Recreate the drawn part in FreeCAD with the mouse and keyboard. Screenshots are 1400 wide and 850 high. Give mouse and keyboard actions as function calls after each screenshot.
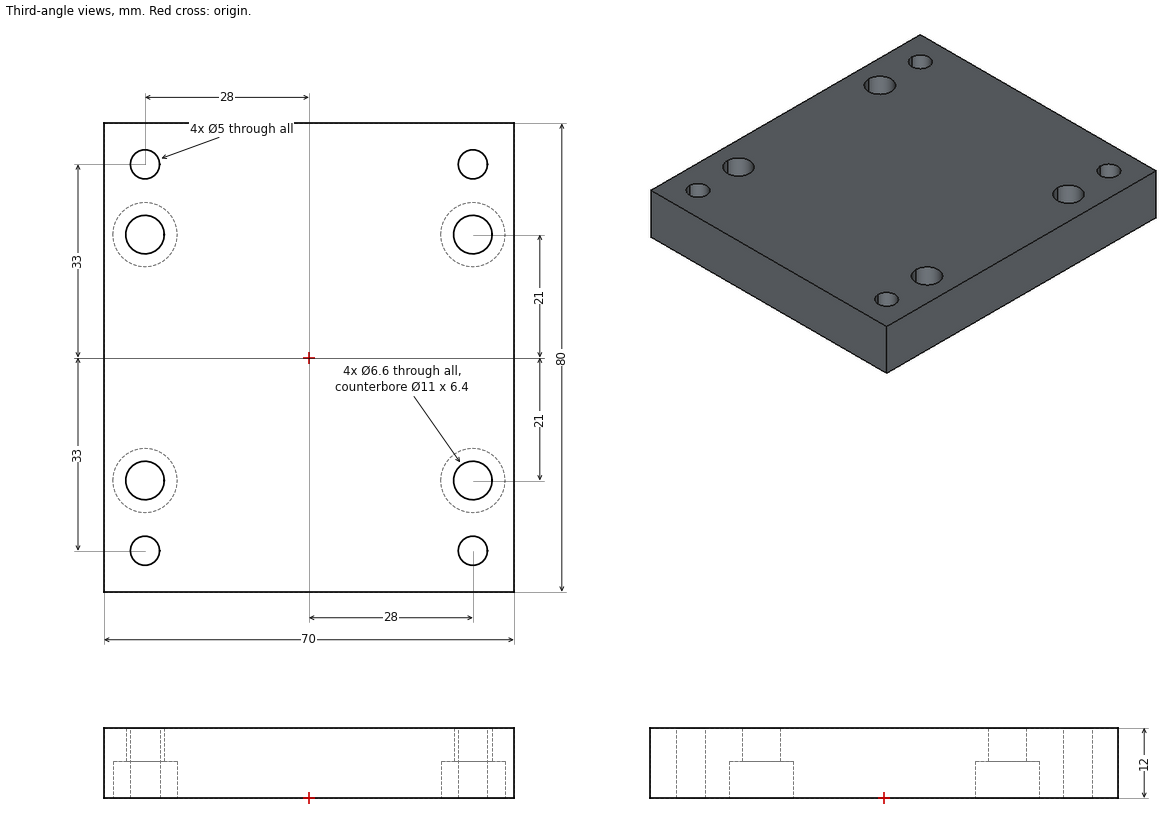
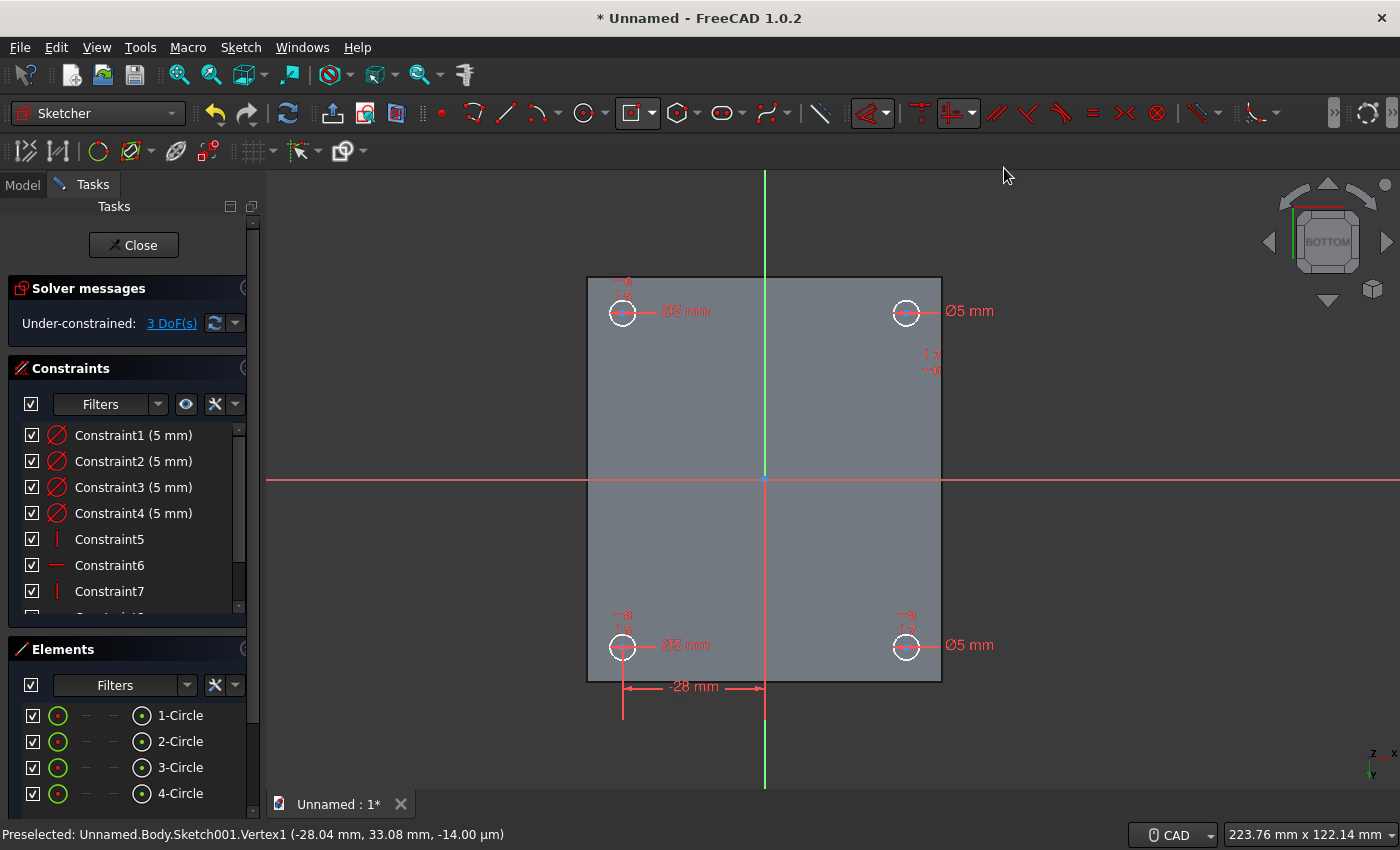
click(623, 647)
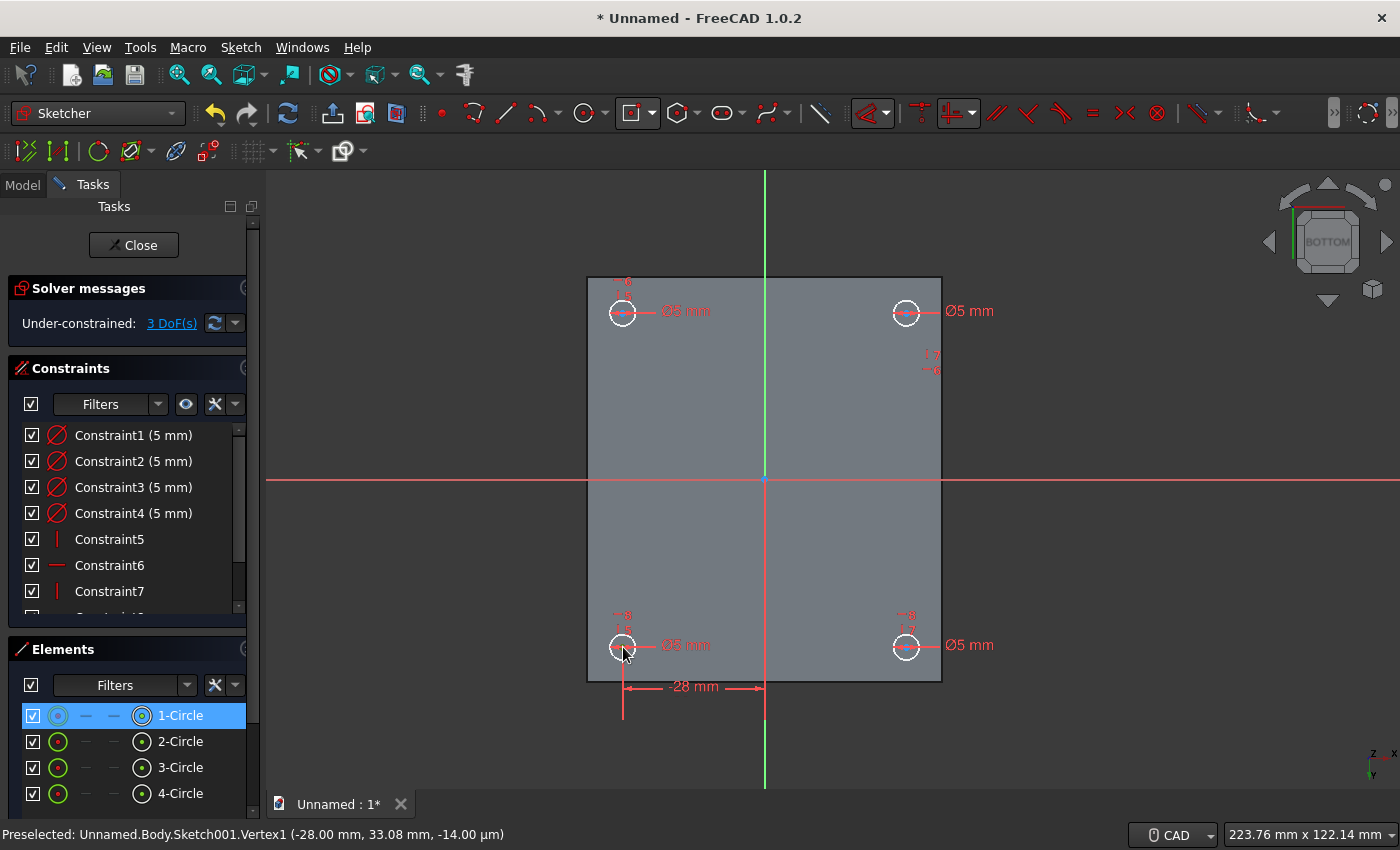
click(888, 114)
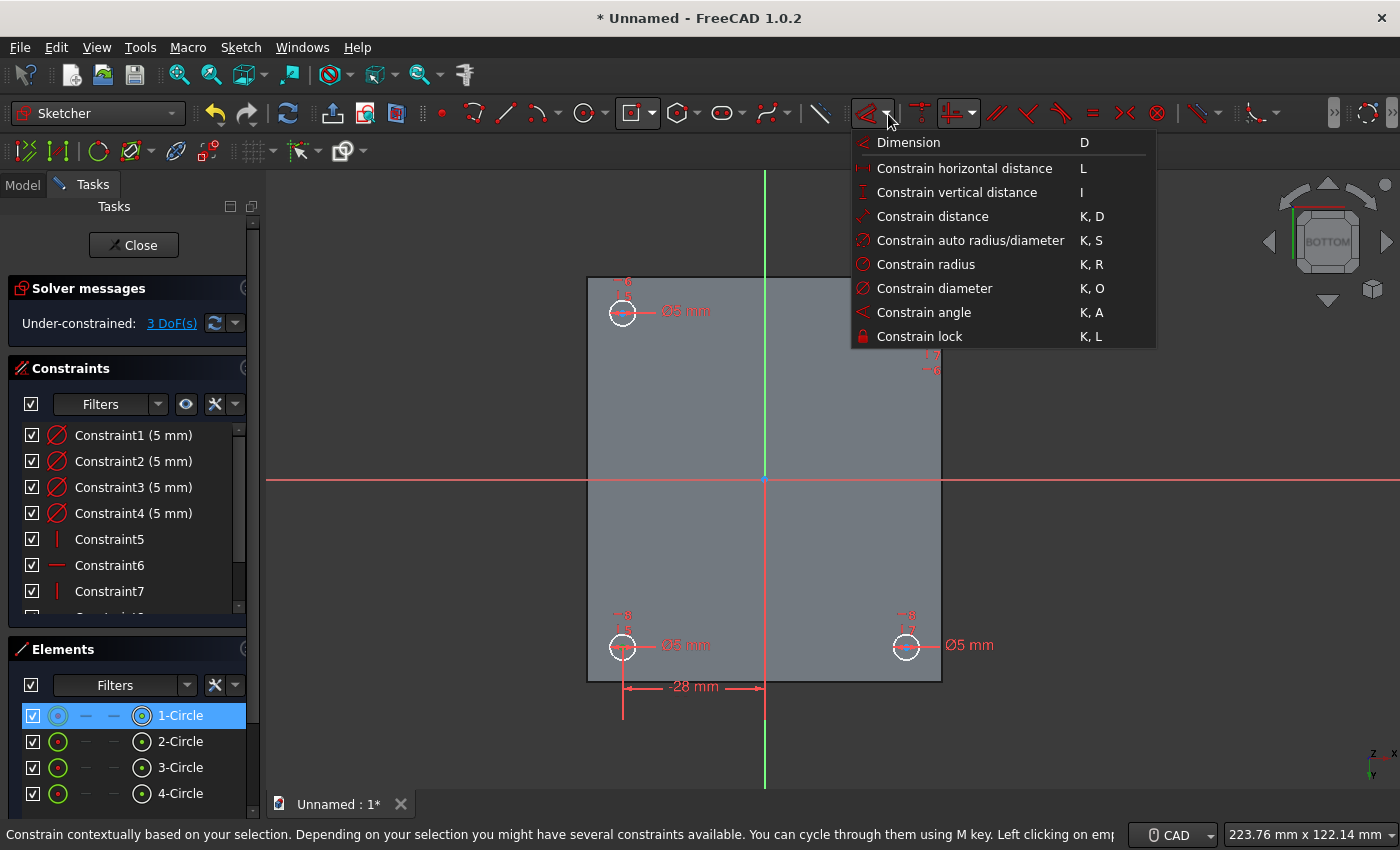
click(1004, 192)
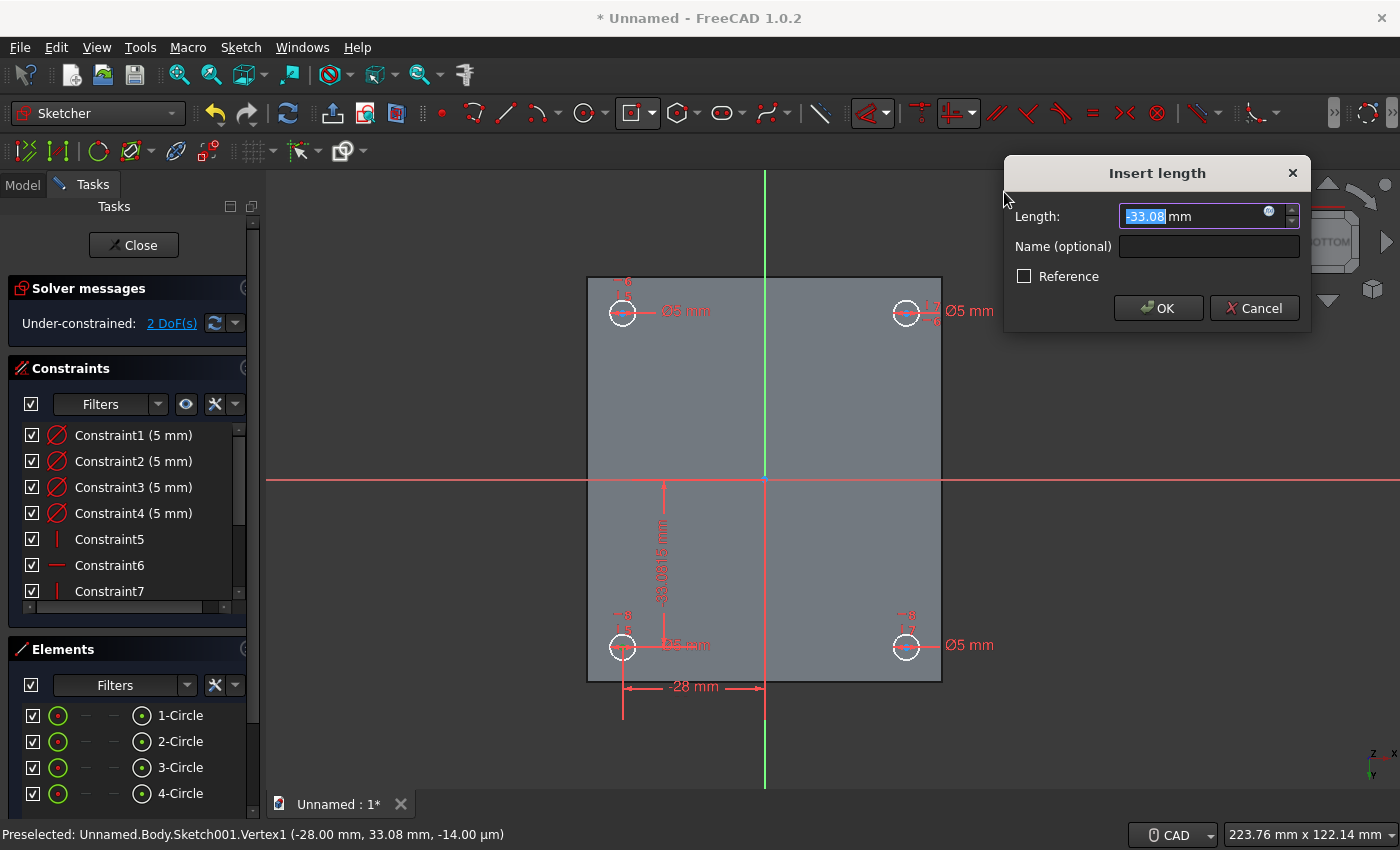
text(-33)
key(Return)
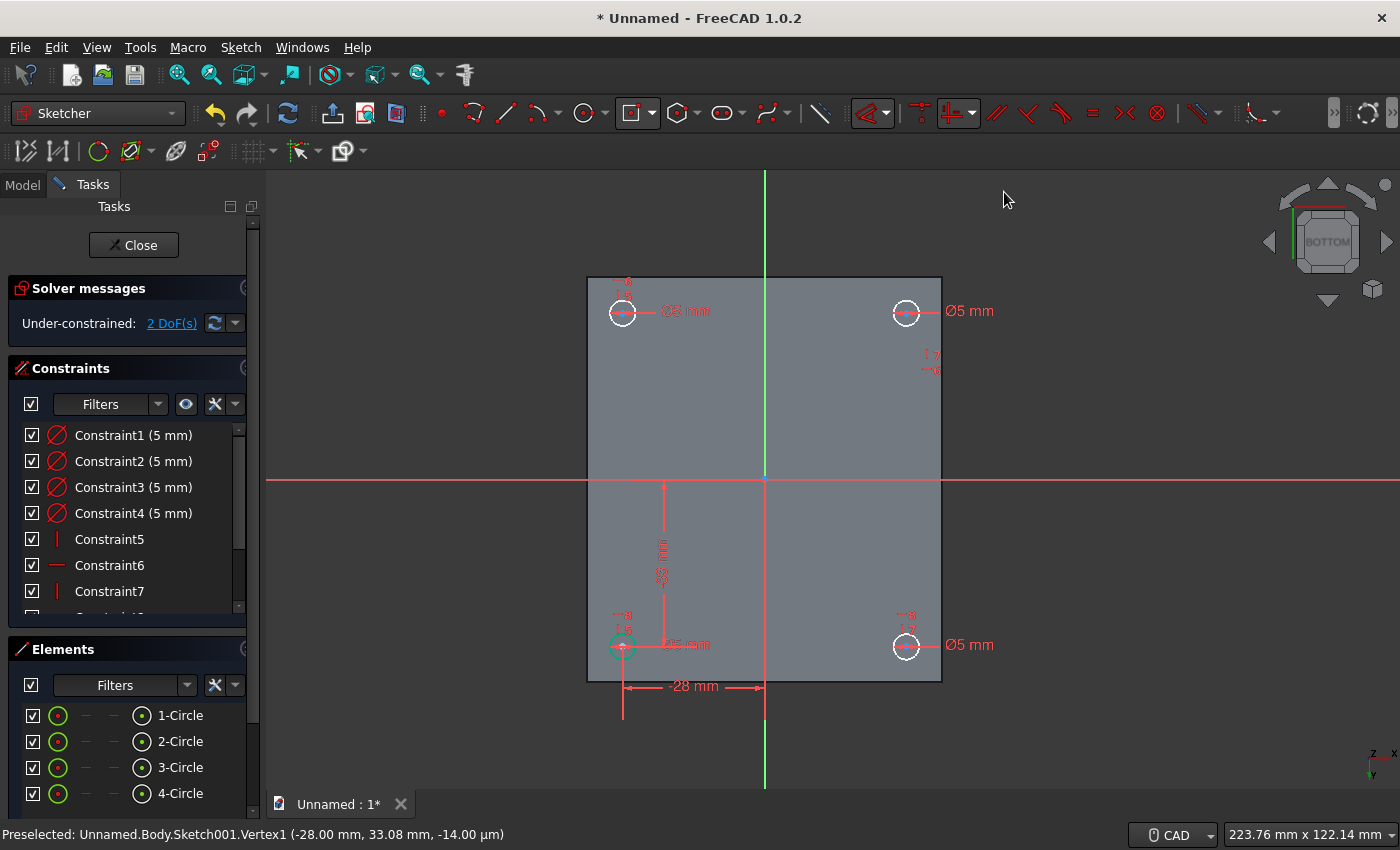
click(623, 313)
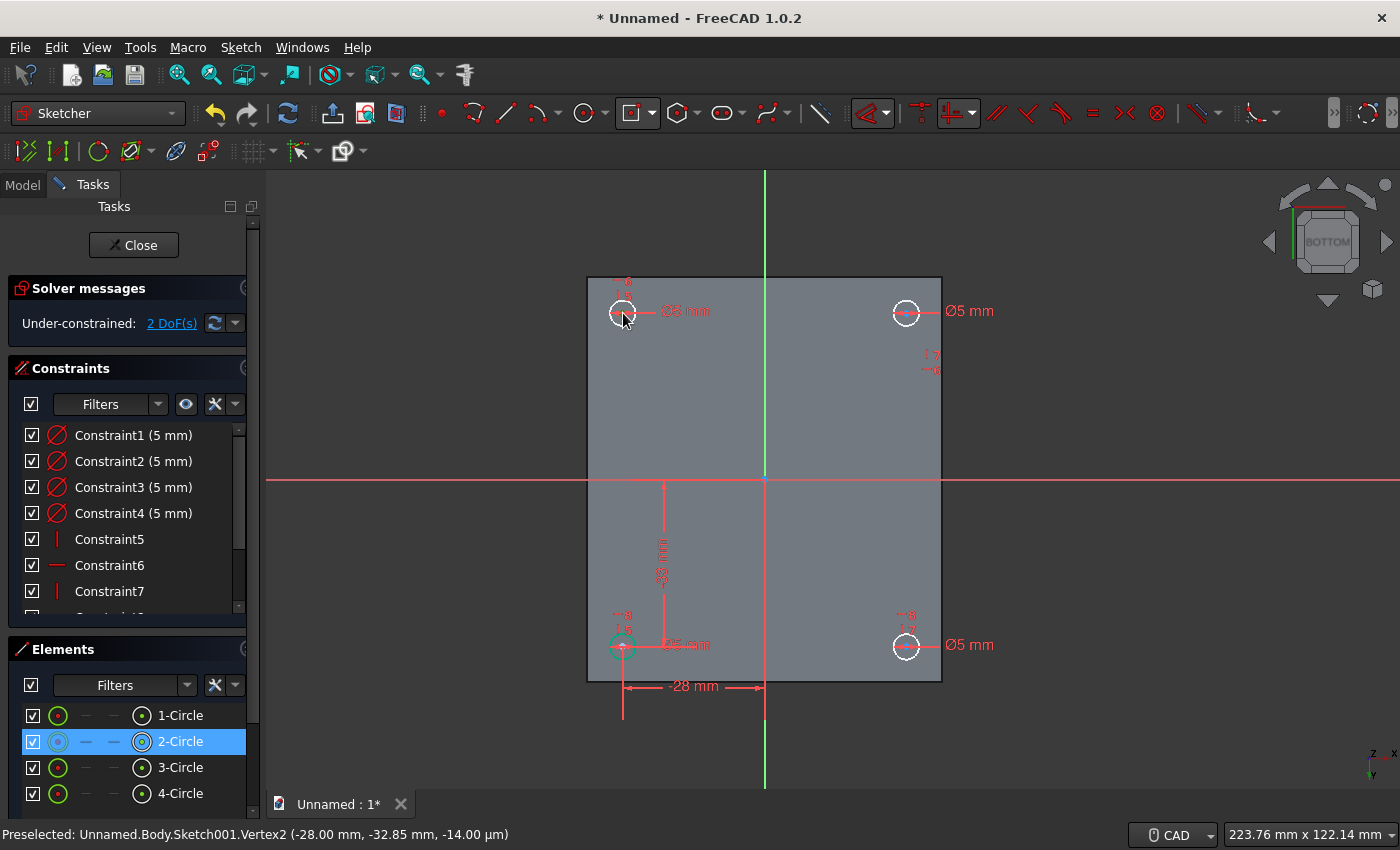
key(i)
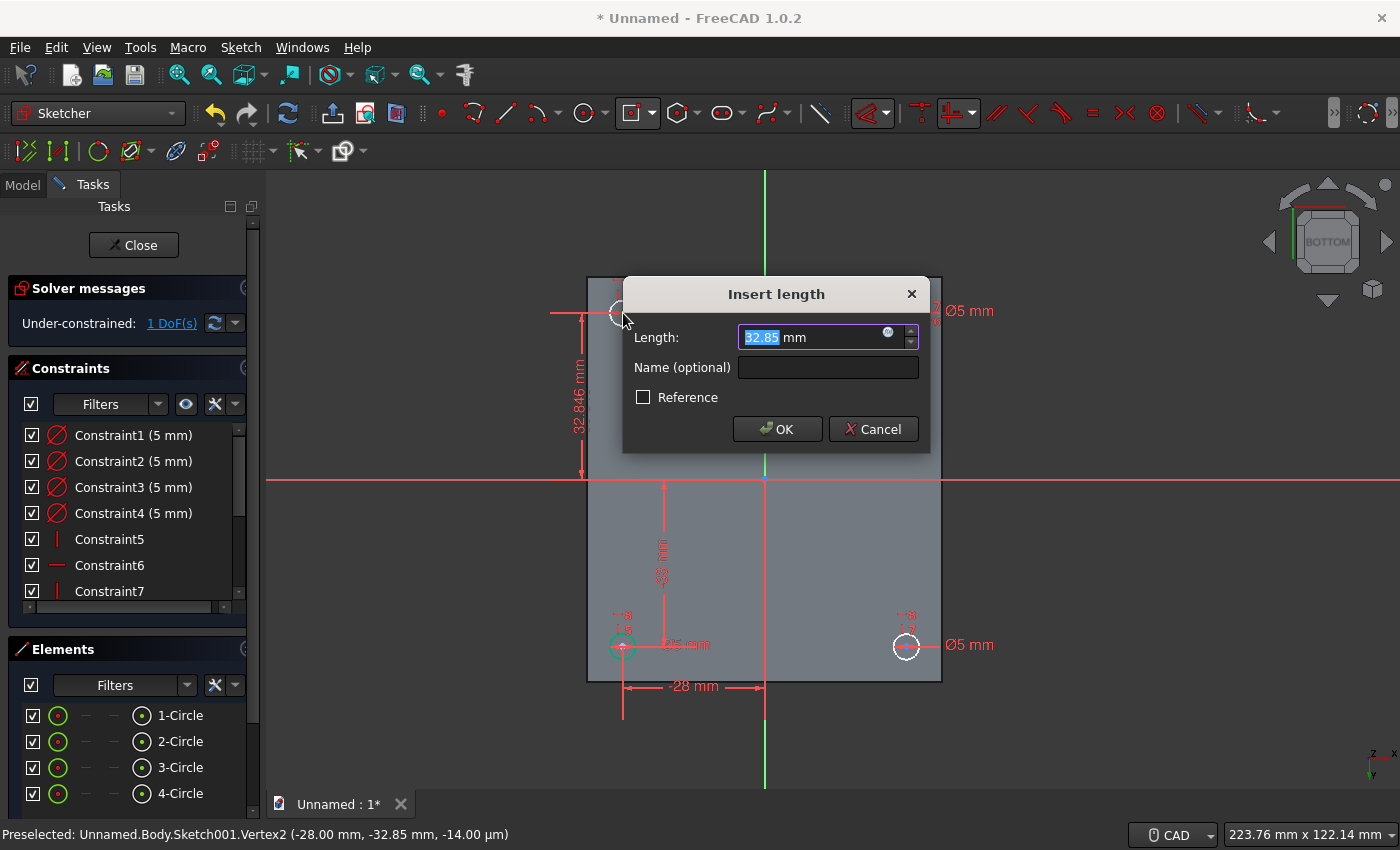
text(33)
key(Return)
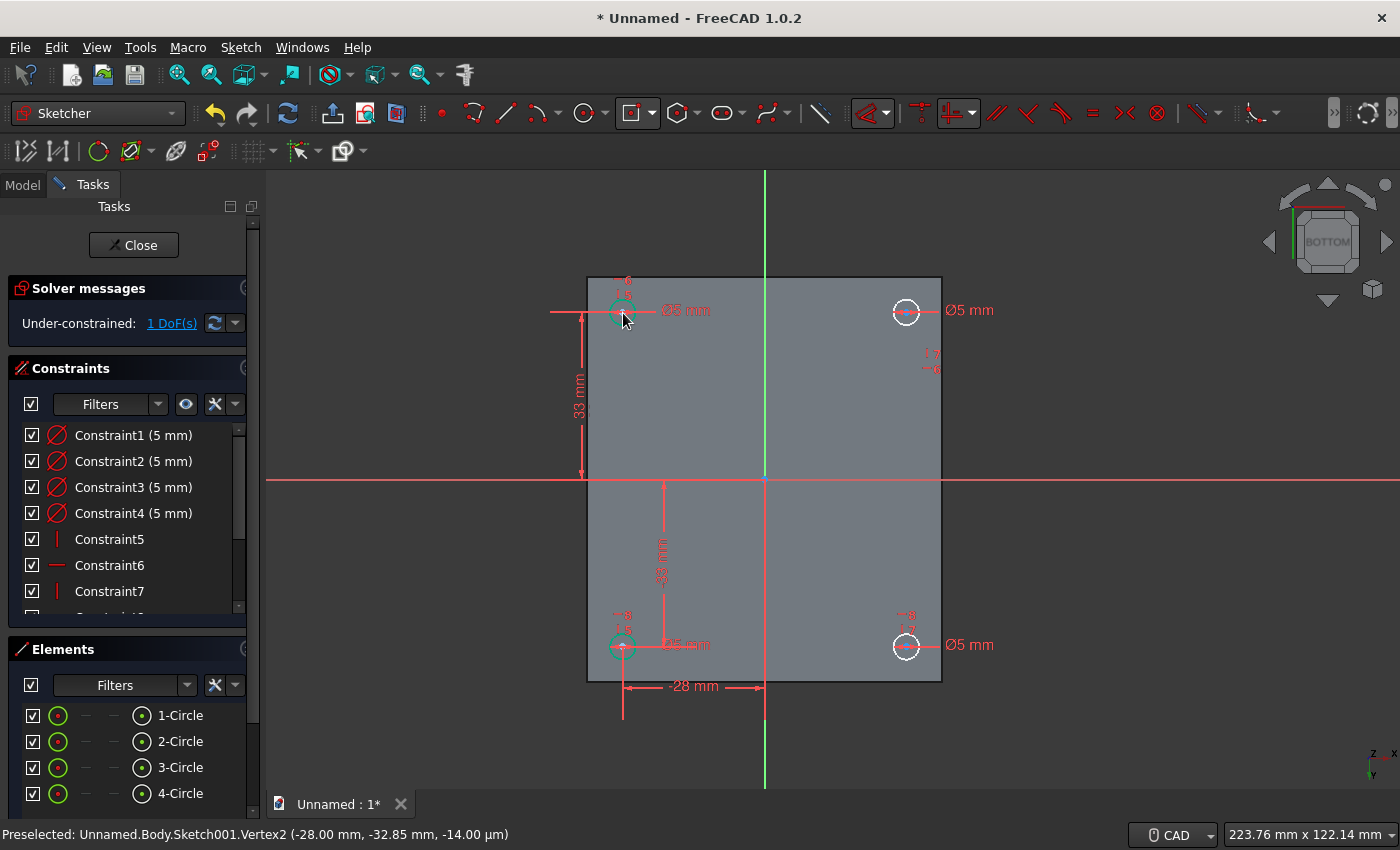
click(906, 312)